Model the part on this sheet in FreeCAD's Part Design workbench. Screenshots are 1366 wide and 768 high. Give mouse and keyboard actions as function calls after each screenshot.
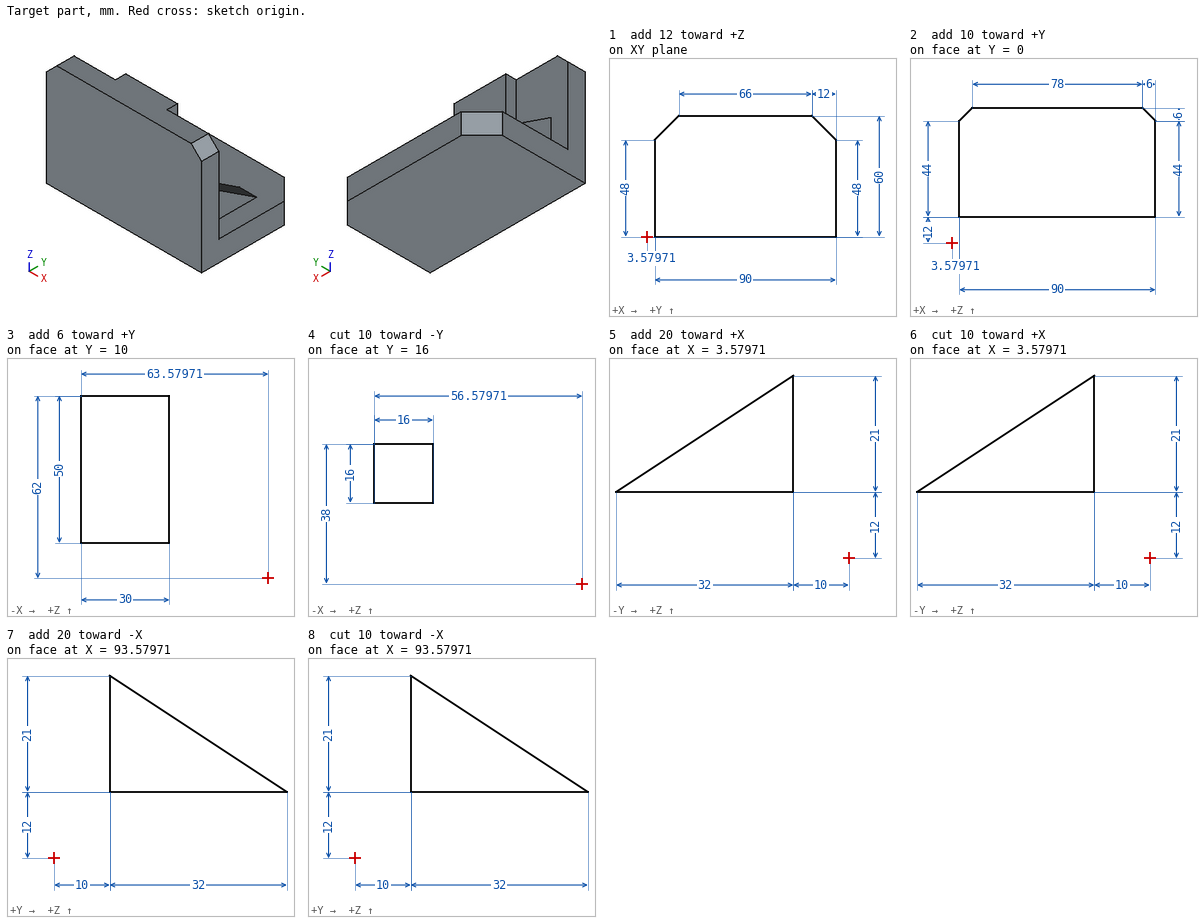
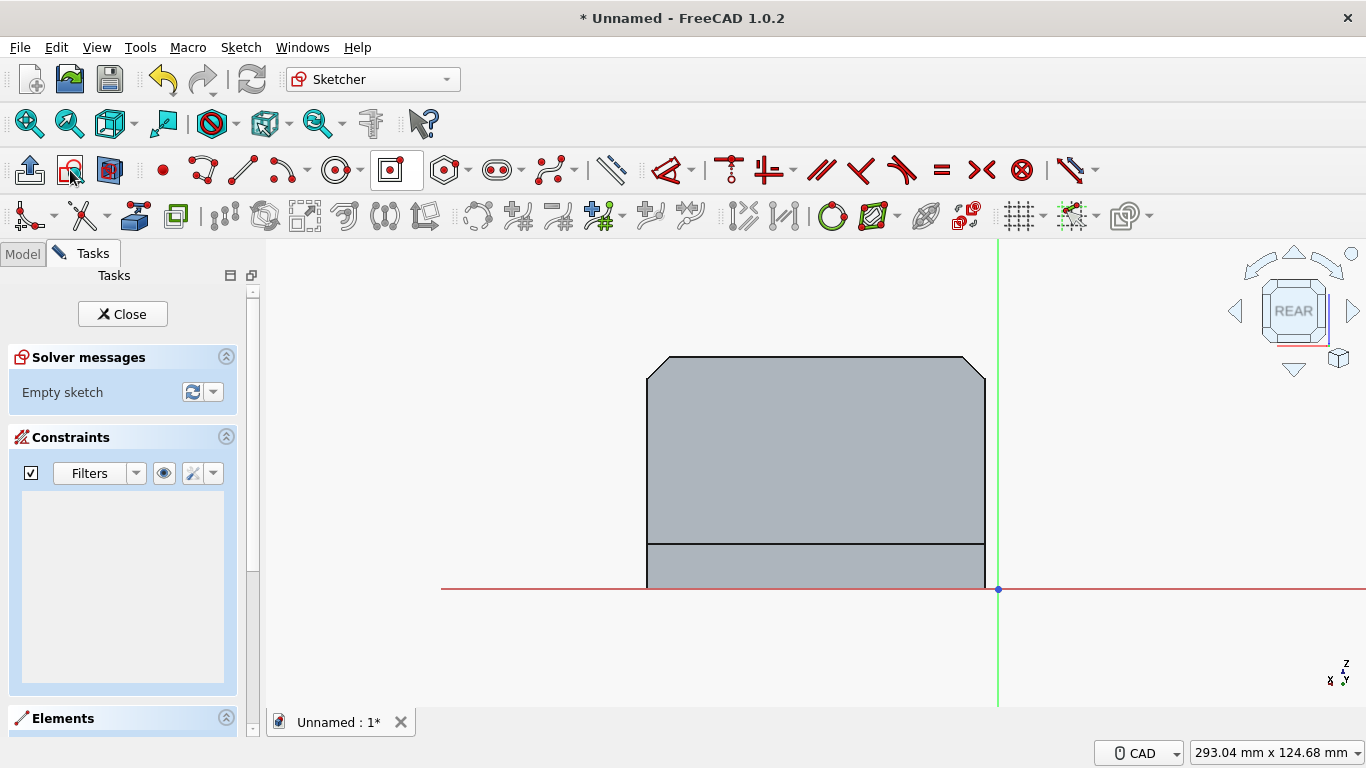
key(g)
key(r)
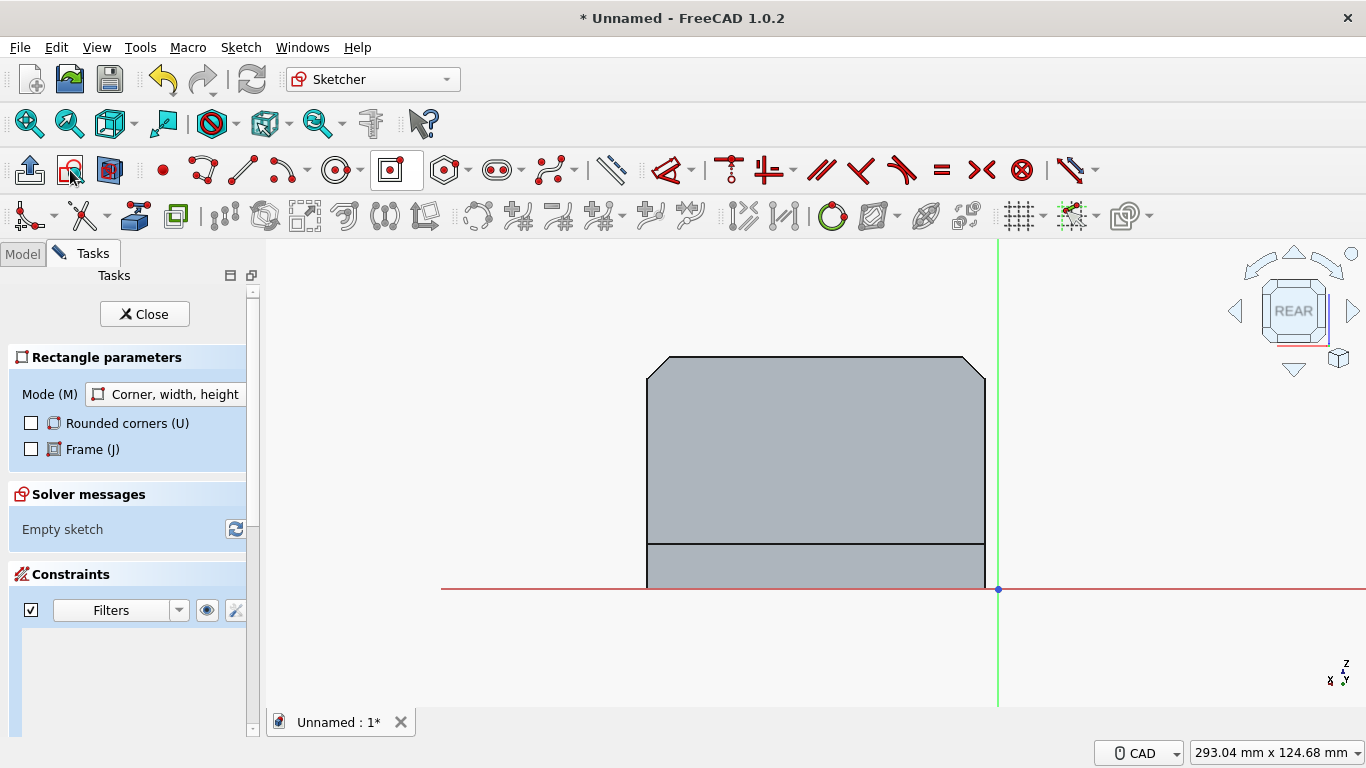
click(760, 357)
click(872, 544)
key(Escape)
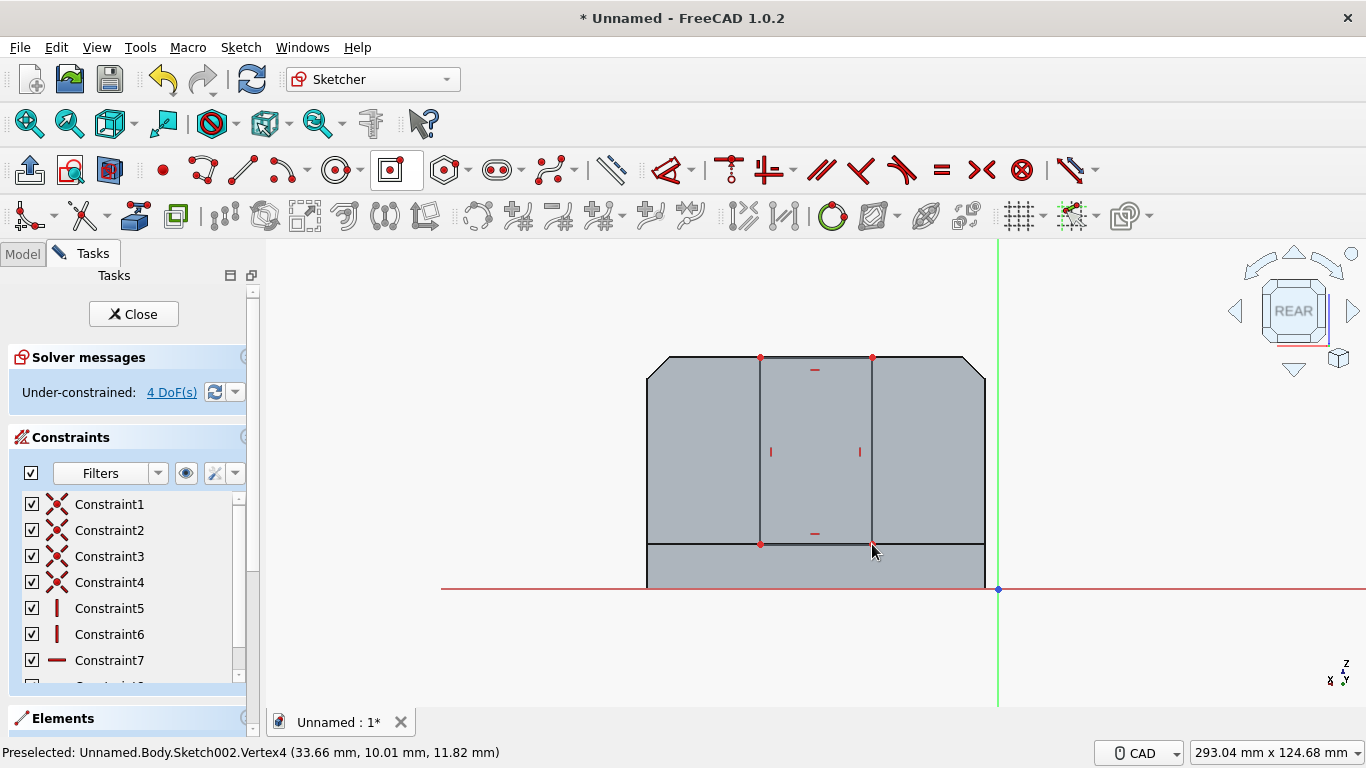
key(d)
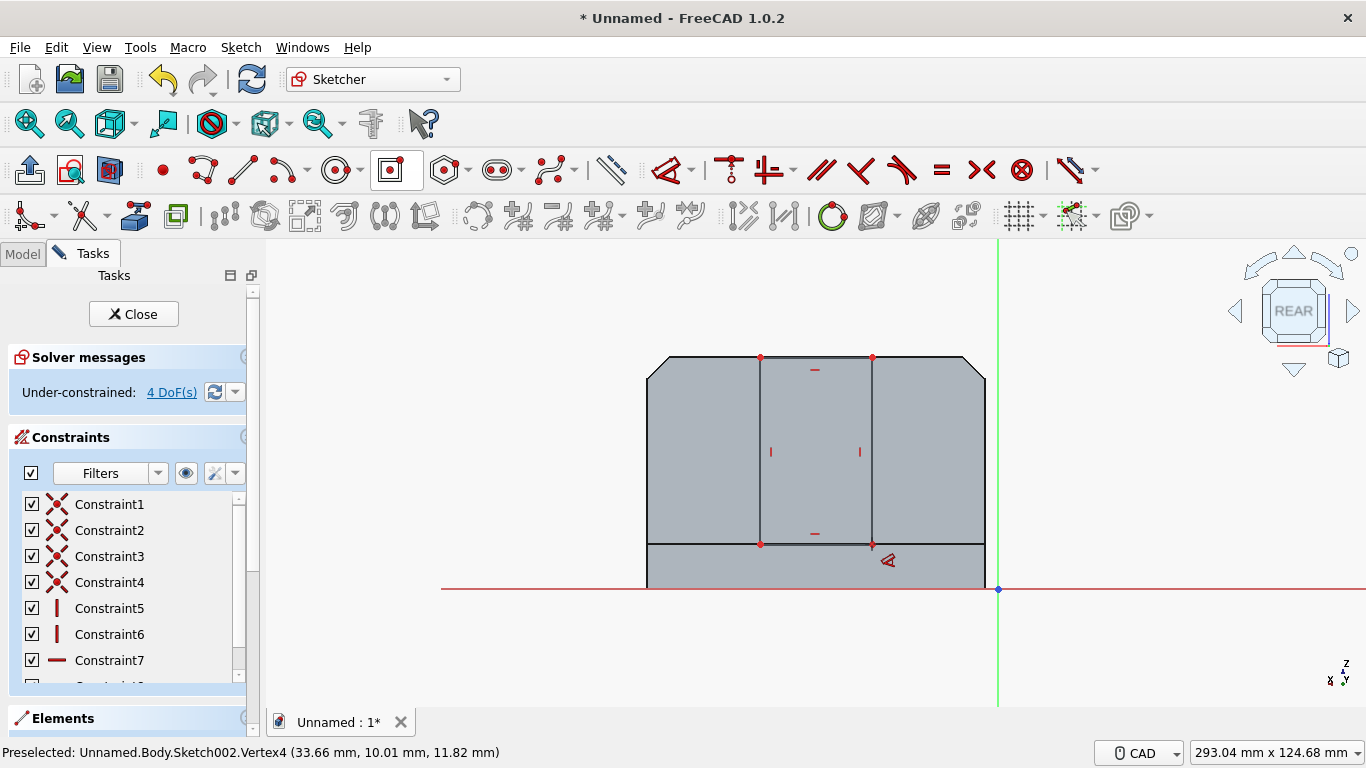
click(760, 414)
click(726, 452)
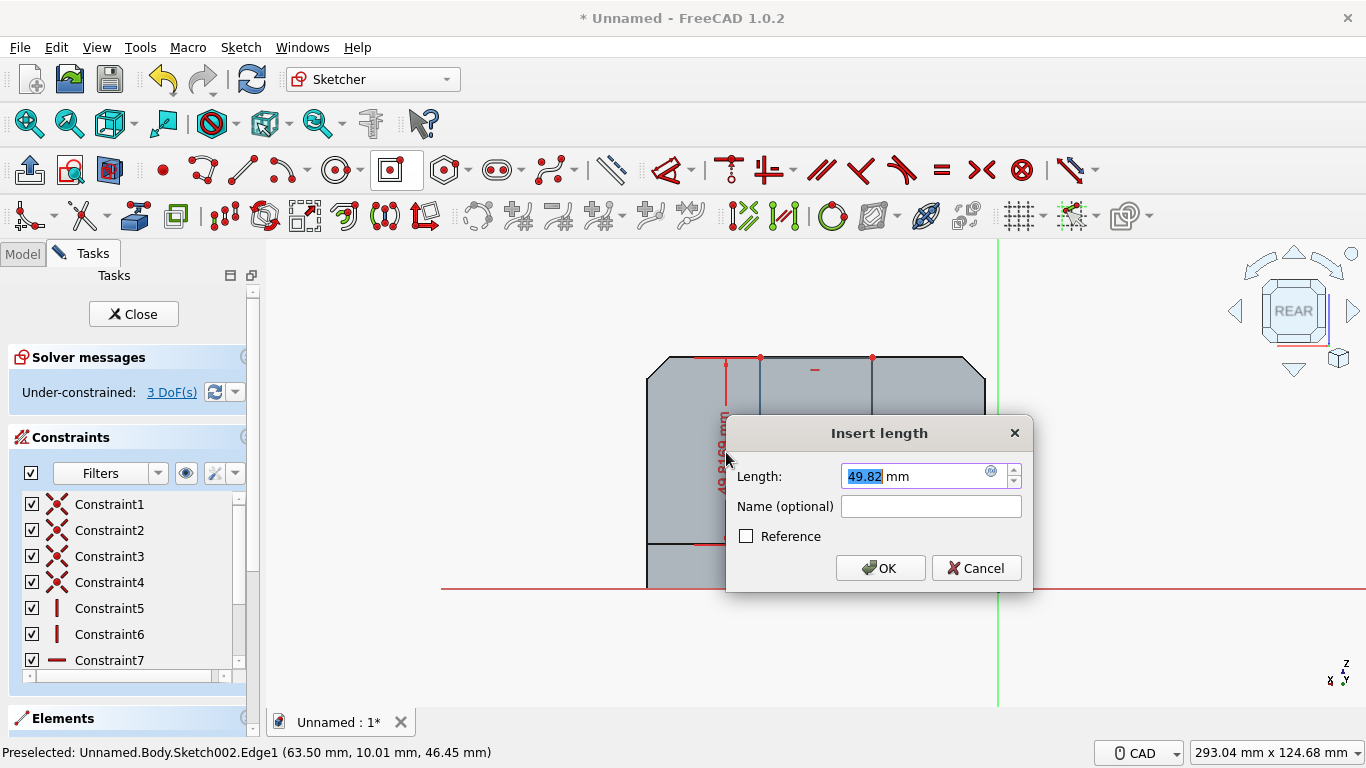
text(50)
key(Return)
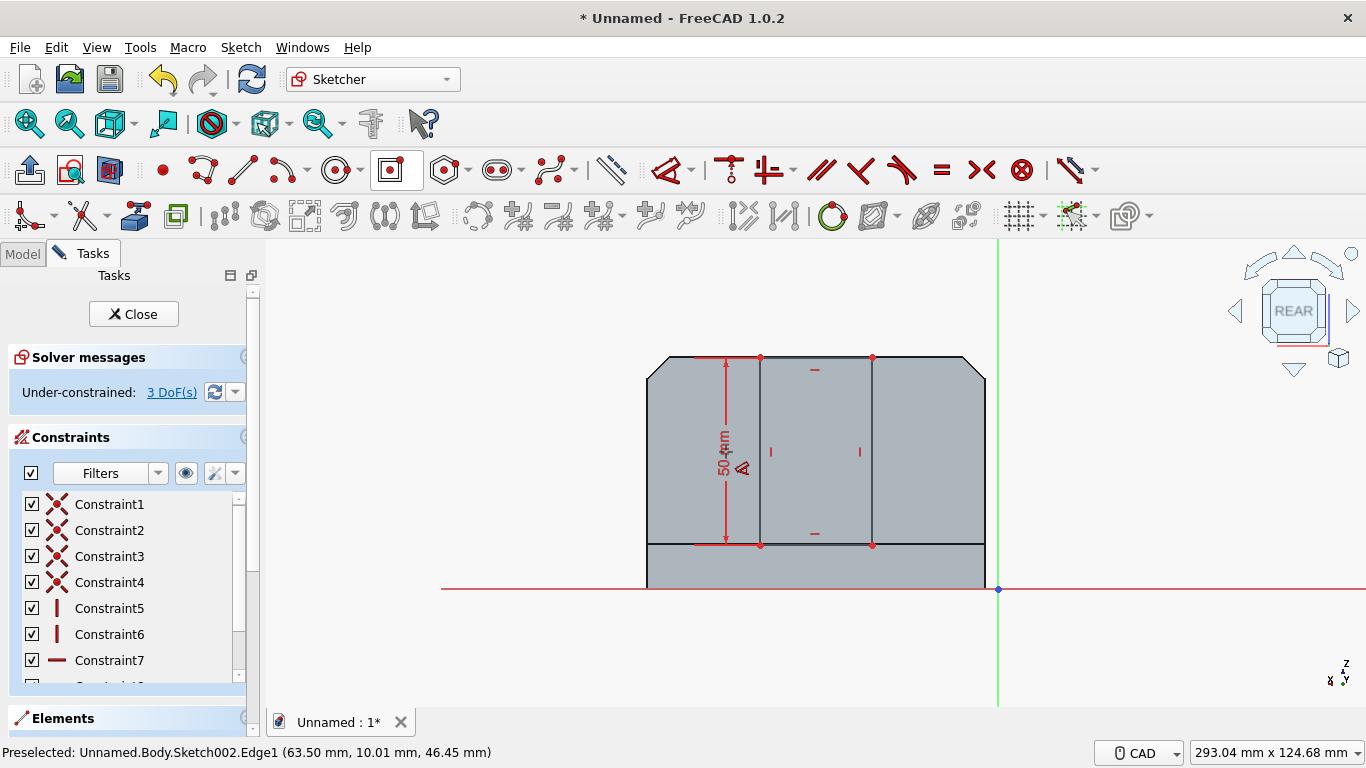
click(794, 545)
click(816, 511)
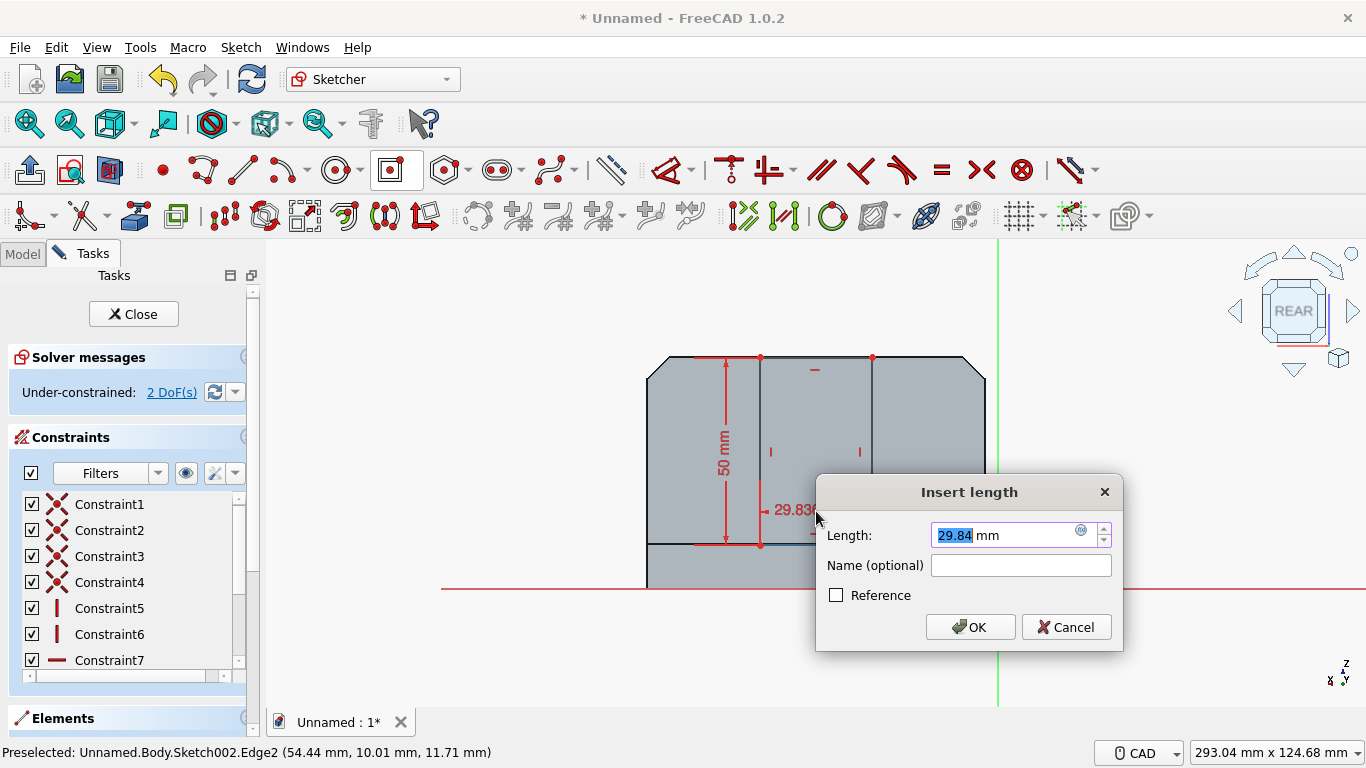
text(30)
key(Return)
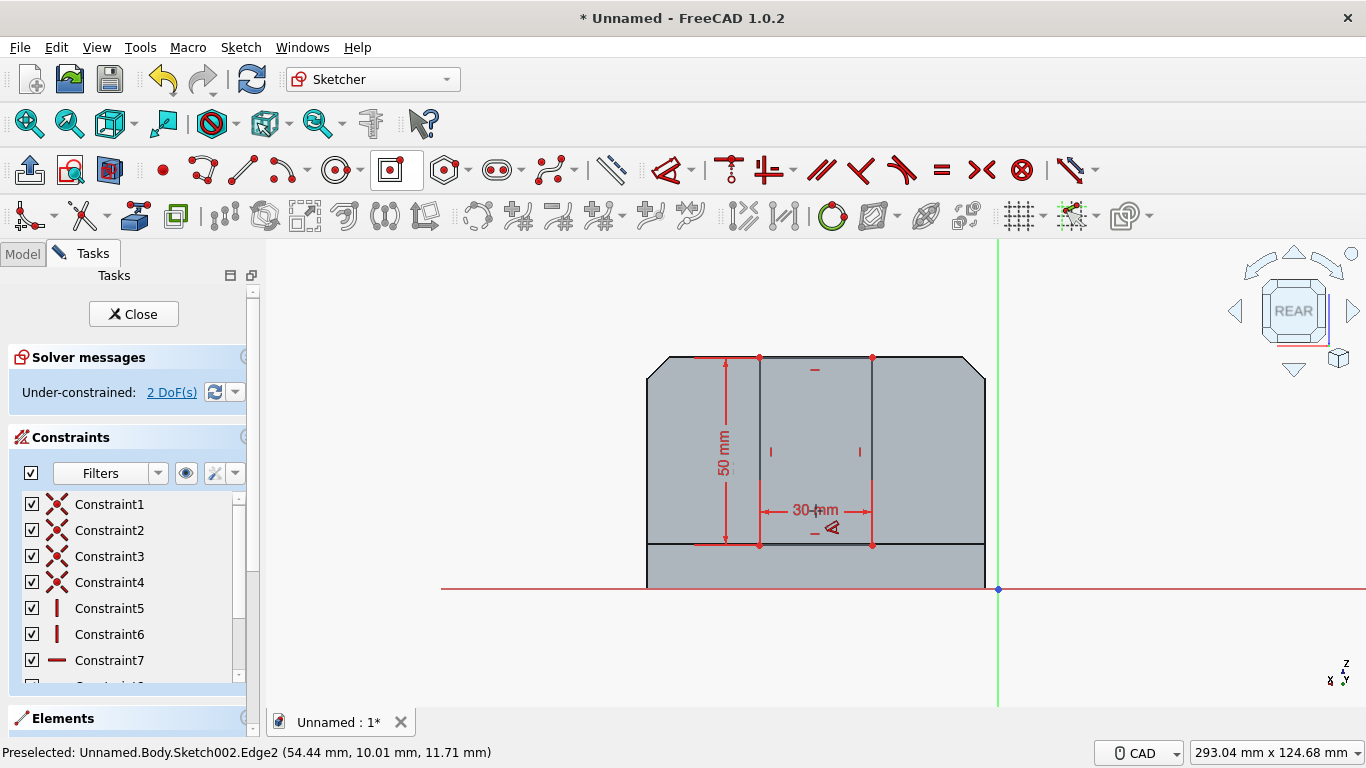
click(760, 358)
click(726, 474)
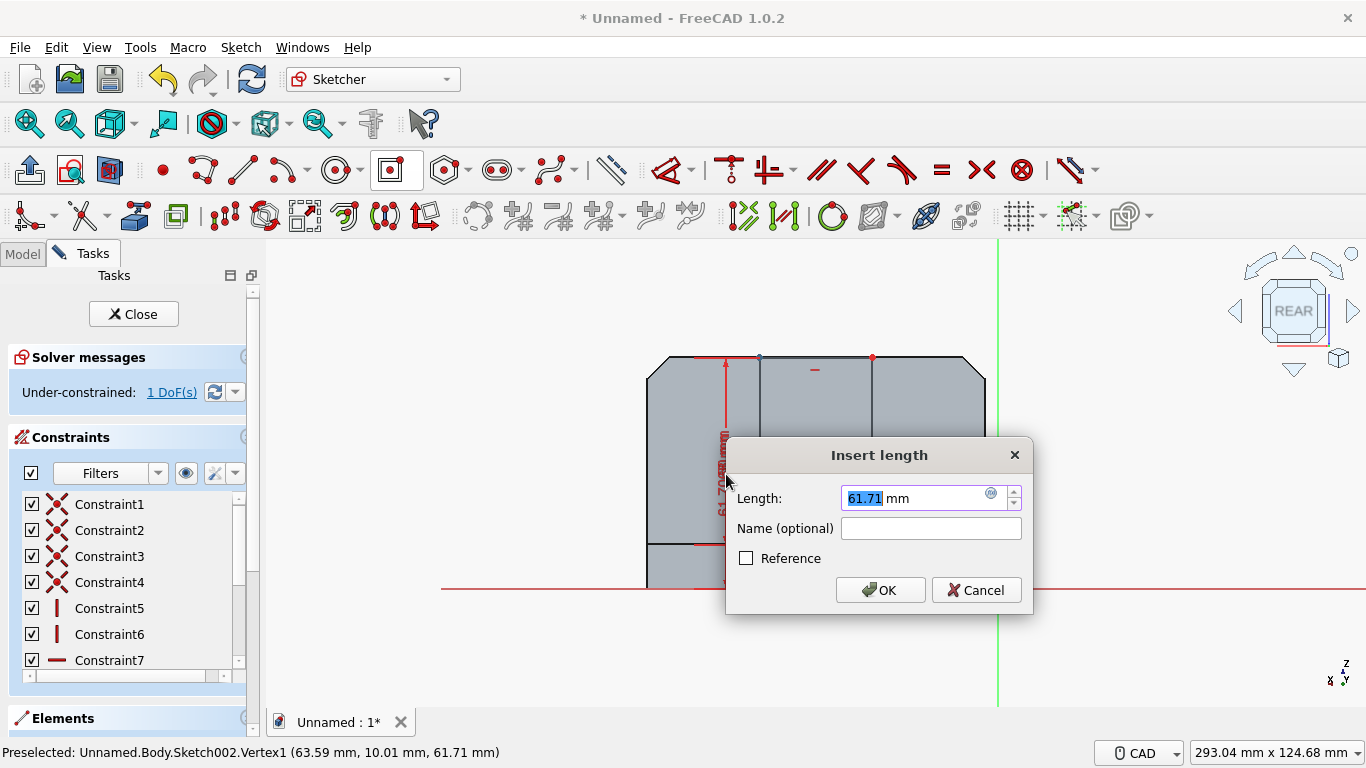
text(62)
key(Return)